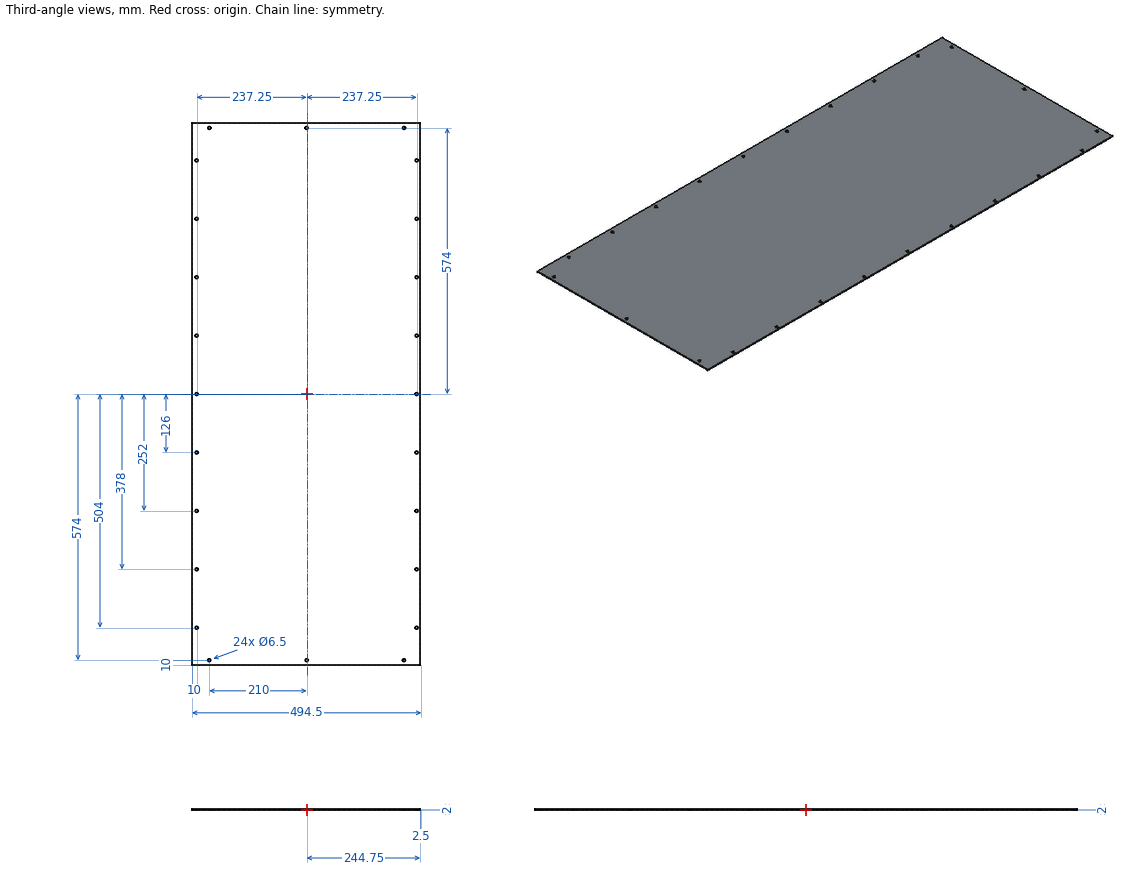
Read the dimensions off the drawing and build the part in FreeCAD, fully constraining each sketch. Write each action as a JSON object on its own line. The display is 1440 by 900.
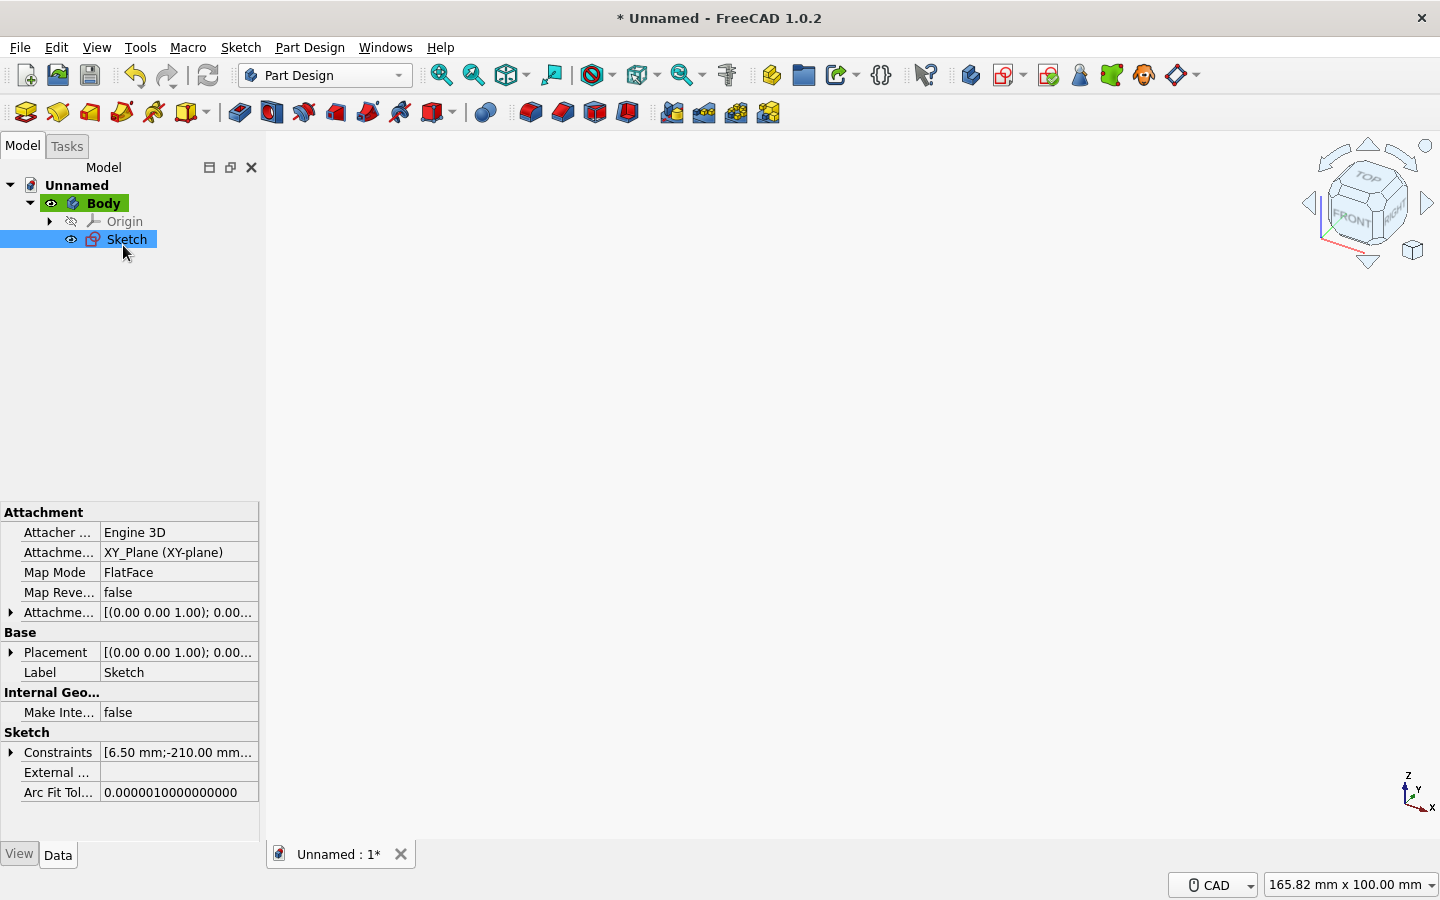
{"action": "left_click", "coordinate": [26, 112]}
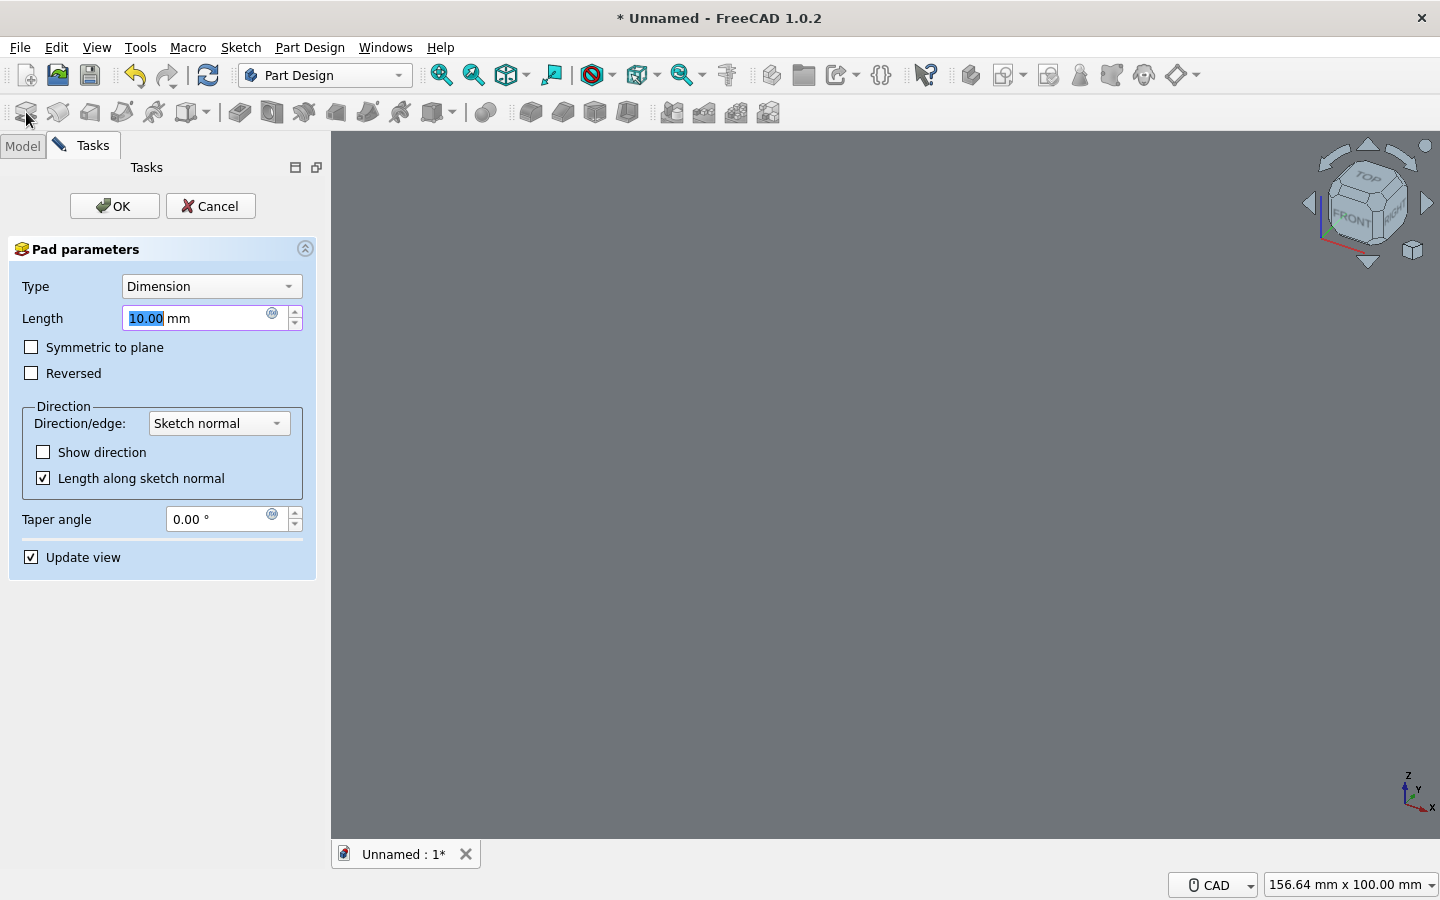
{"action": "type", "text": "2"}
{"action": "key", "text": "Tab"}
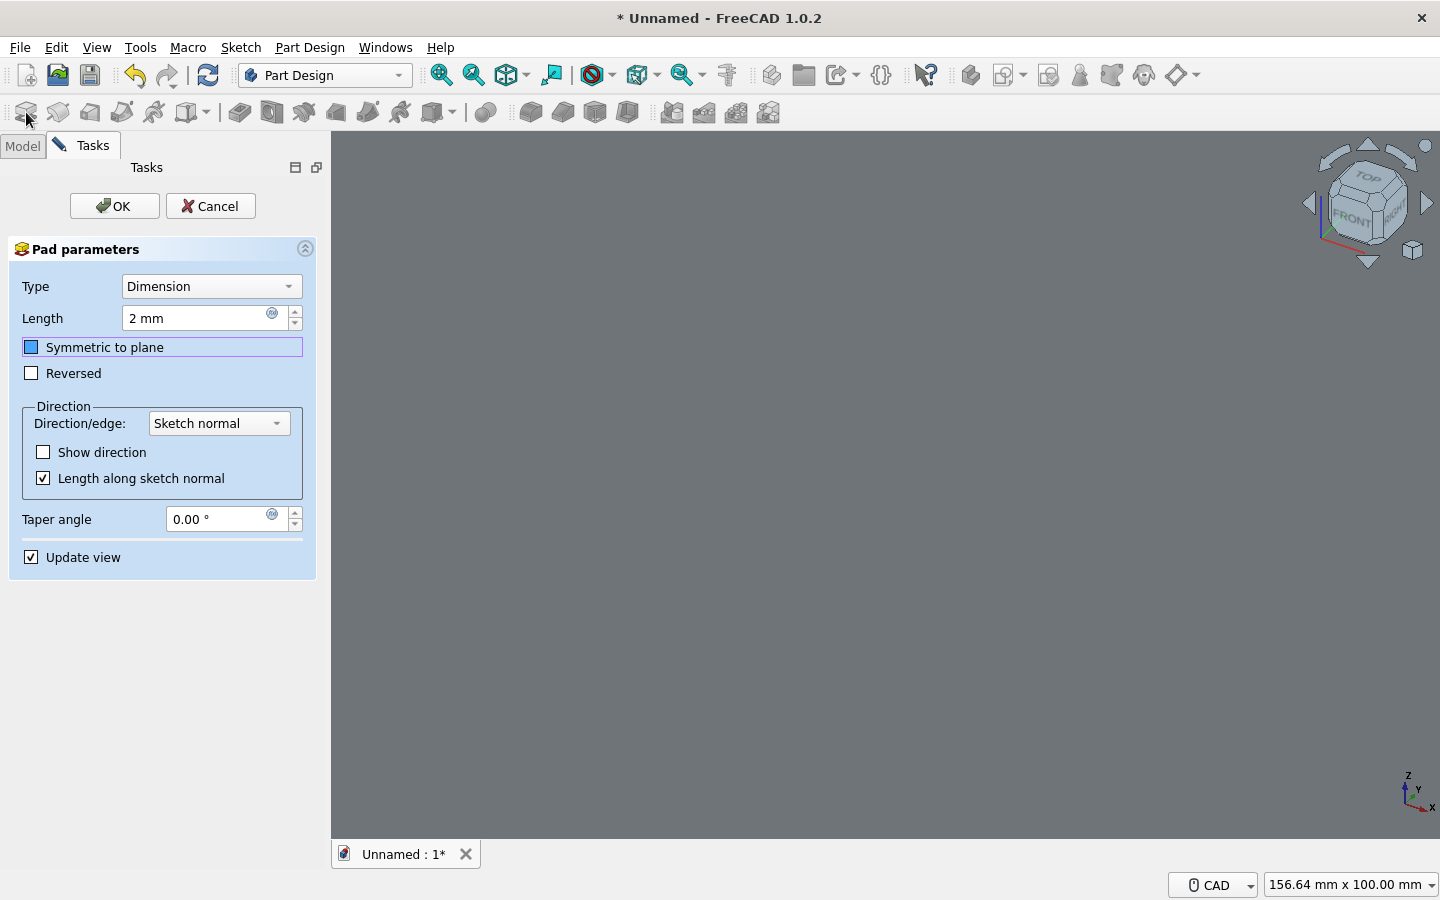
{"action": "left_click", "coordinate": [115, 206]}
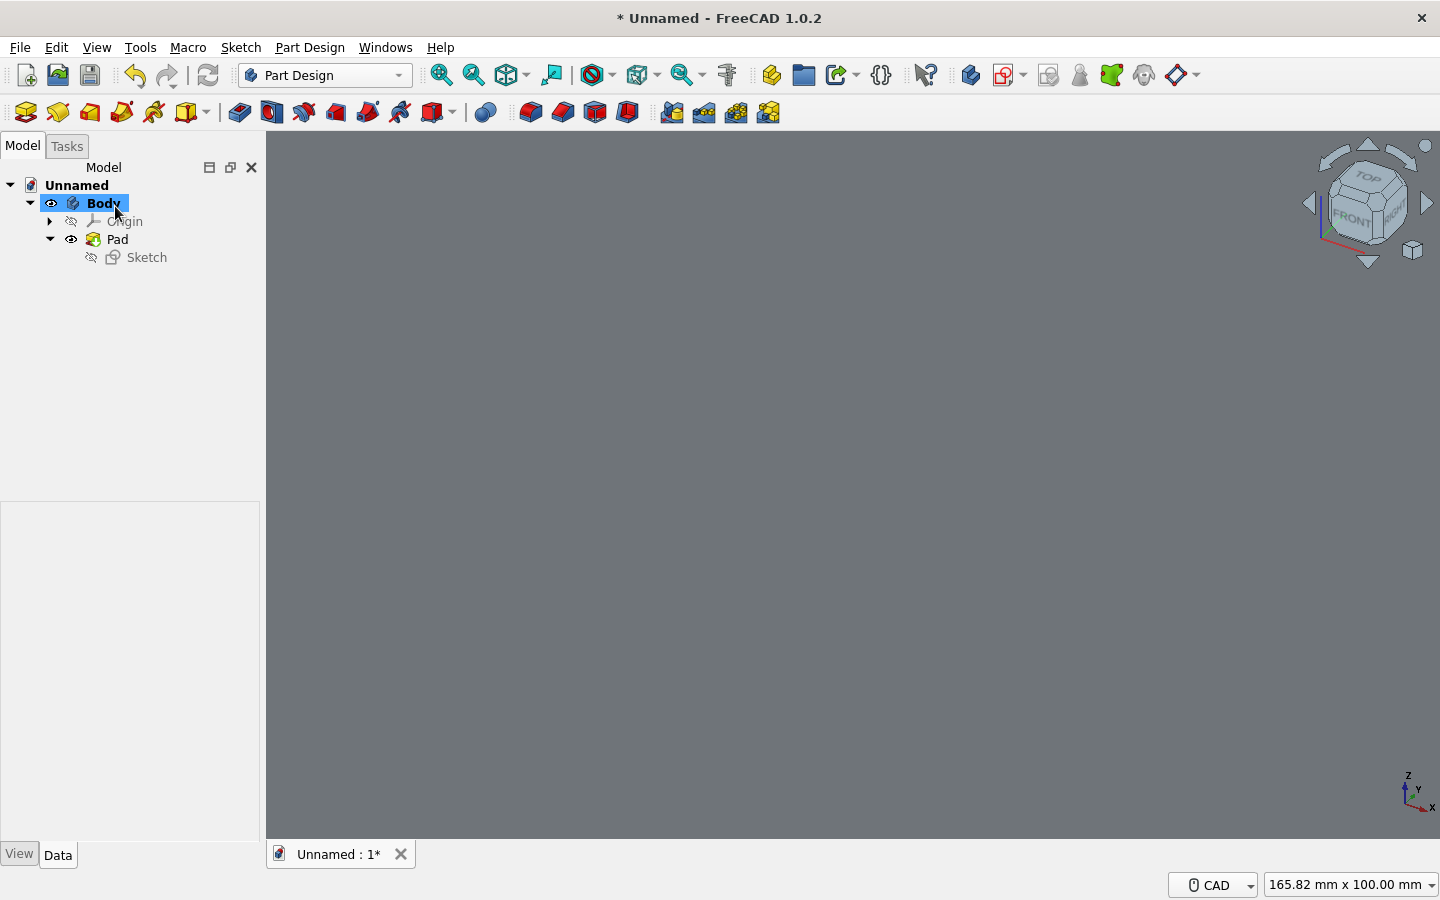
{"action": "key", "text": "v f"}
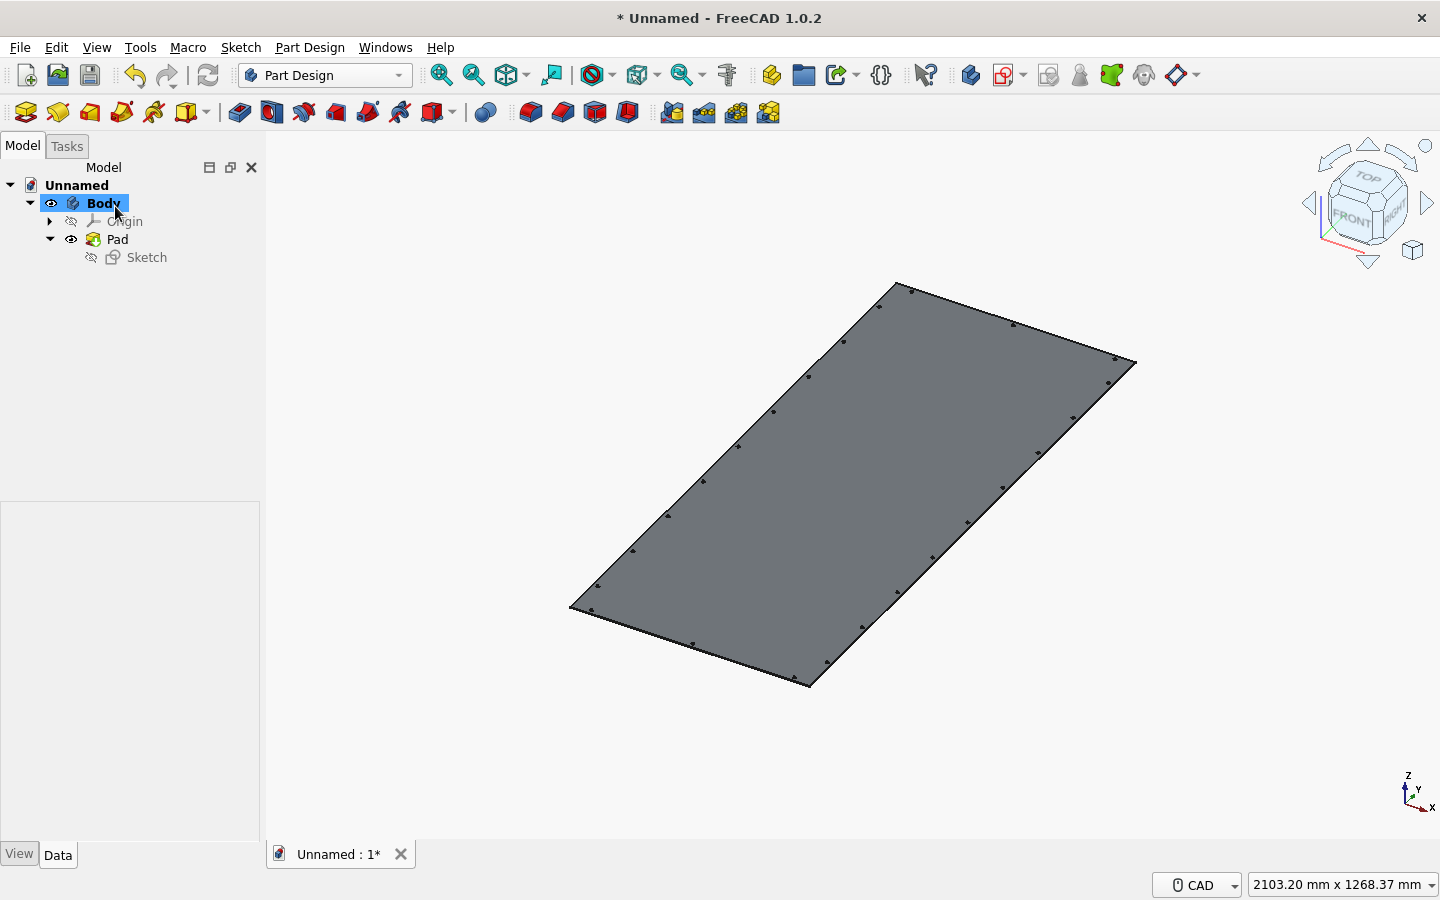
{"action": "scroll", "coordinate": [792, 680], "scroll_direction": "up", "scroll_amount": 15}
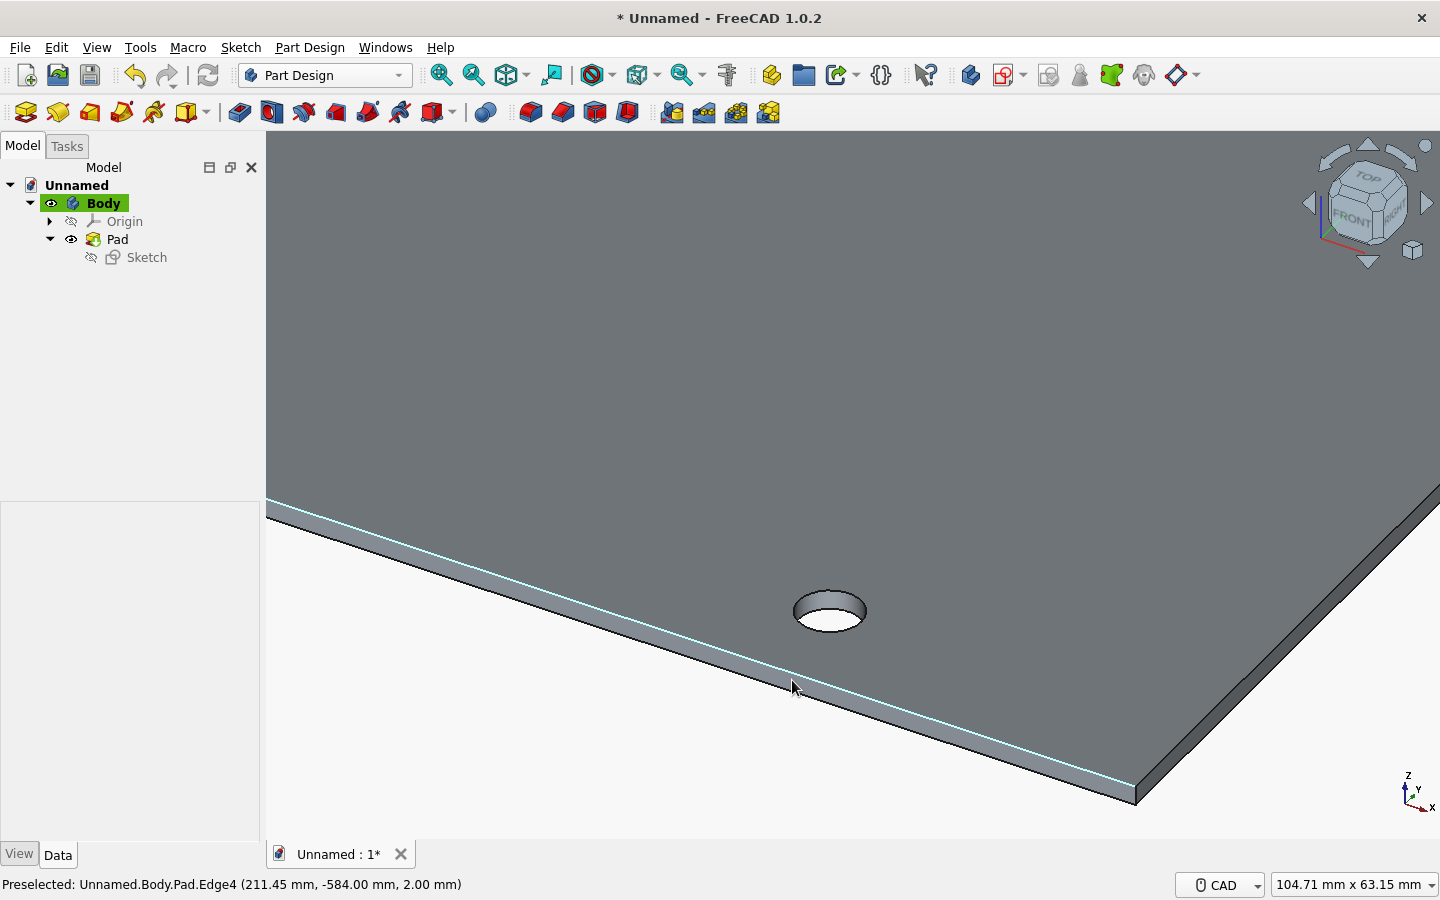
{"action": "key", "text": "v f"}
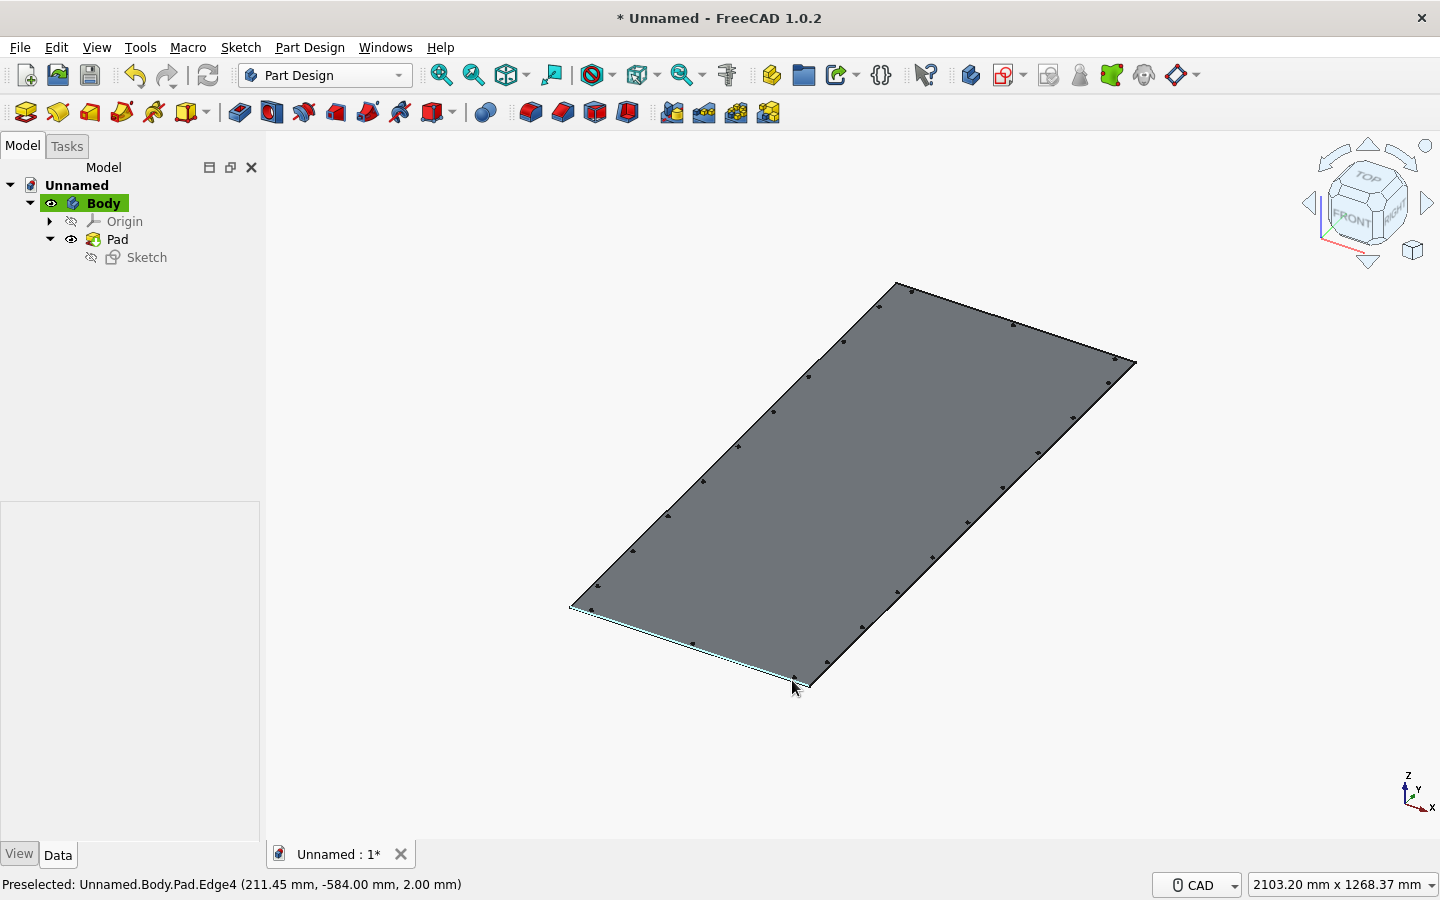
{"action": "key", "text": "0"}